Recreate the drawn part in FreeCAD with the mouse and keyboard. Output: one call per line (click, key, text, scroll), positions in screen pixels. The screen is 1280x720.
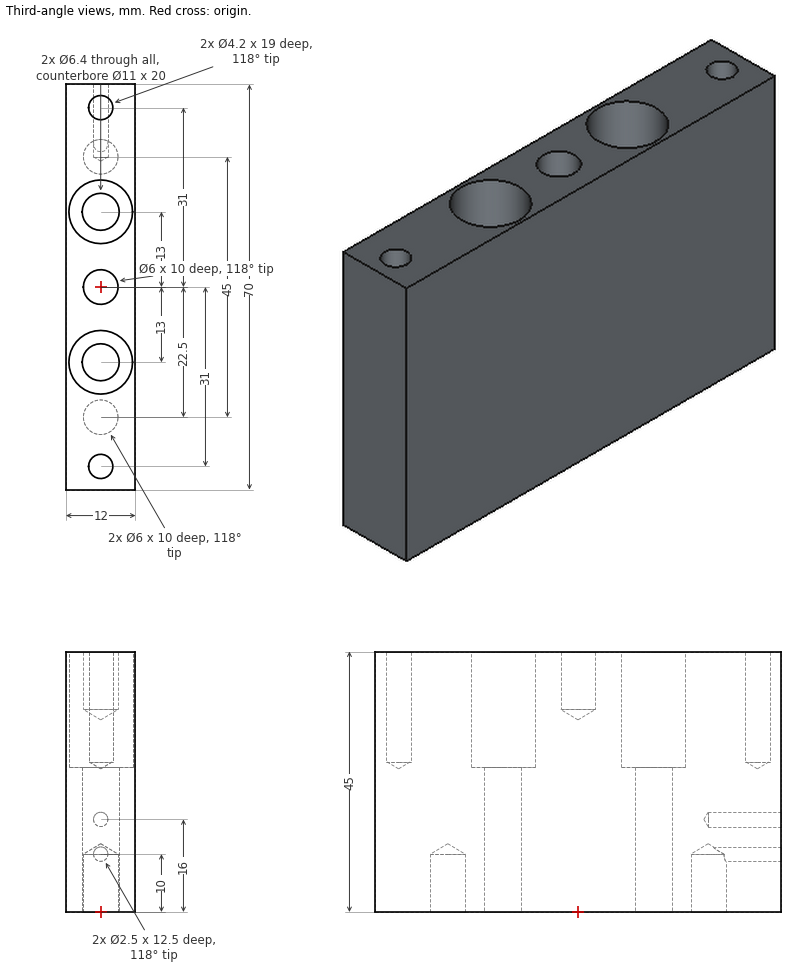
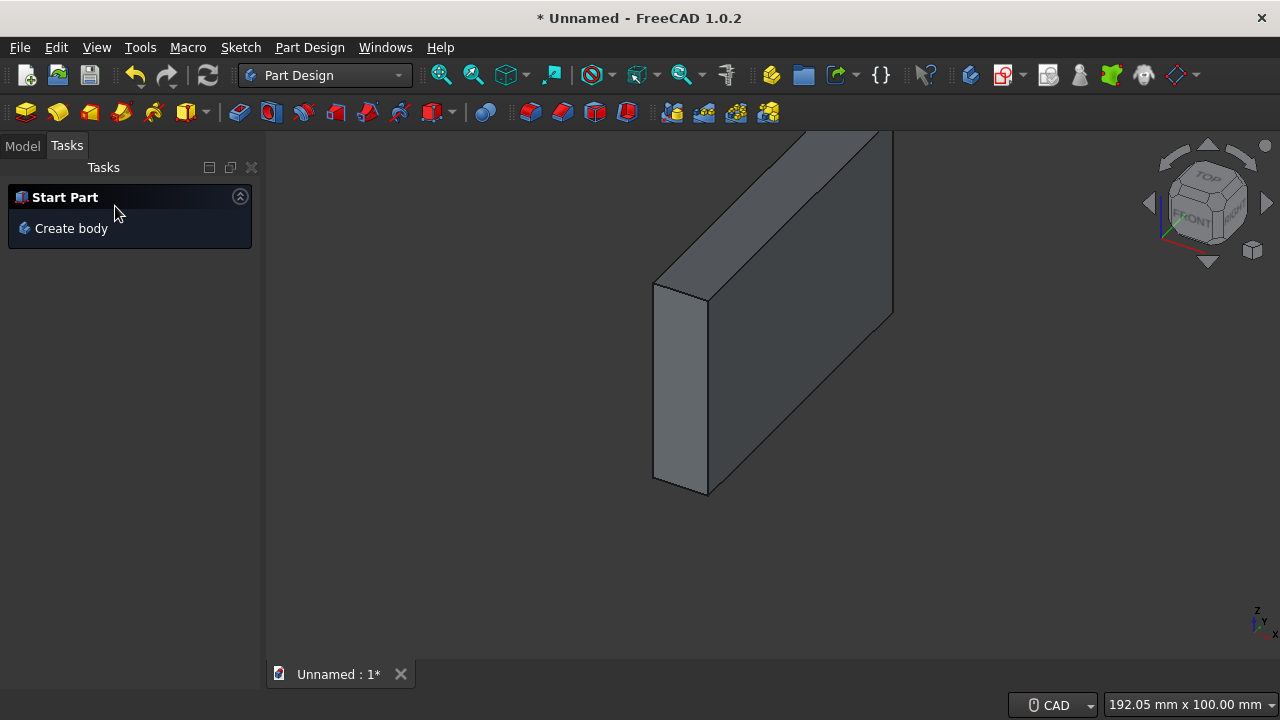
click(442, 76)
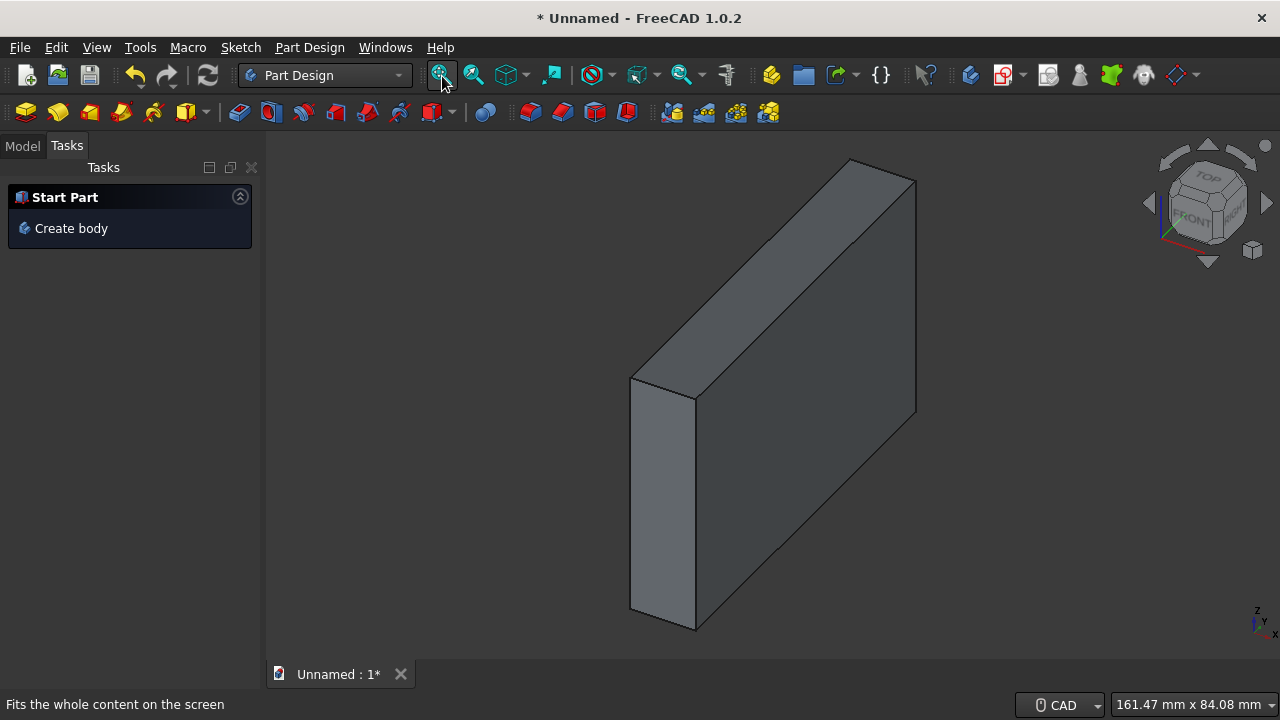
key(4)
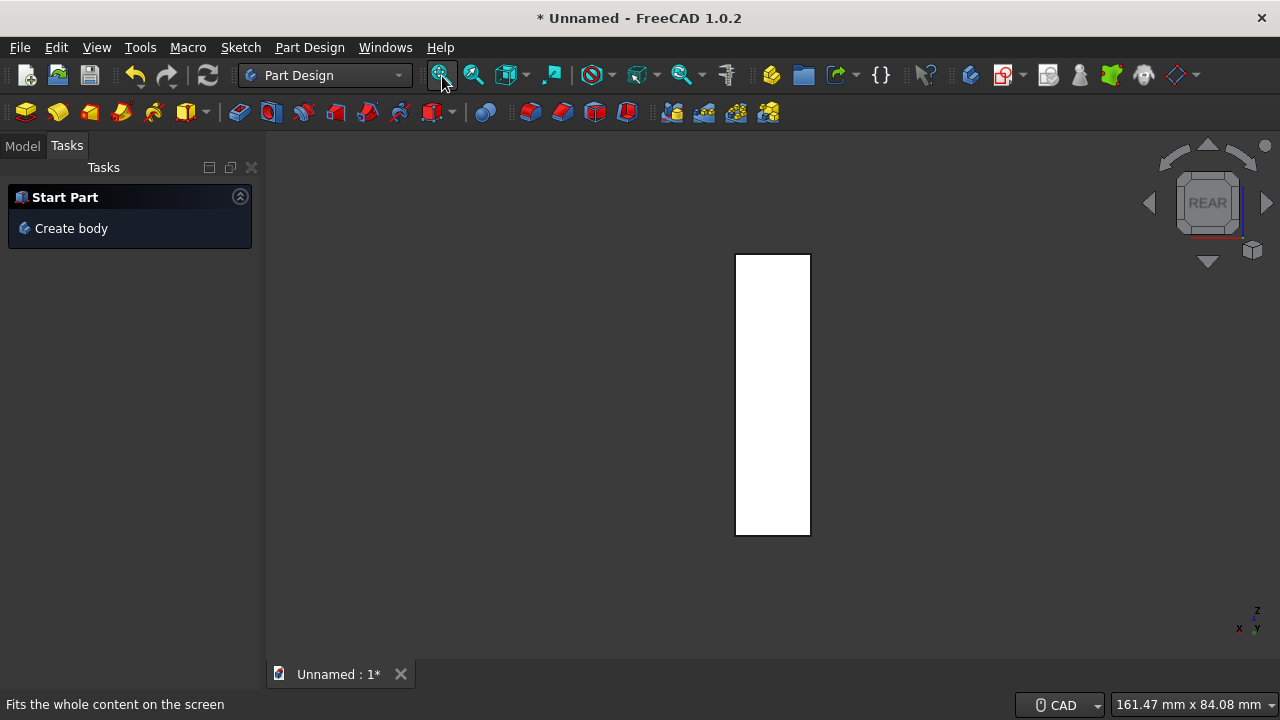
click(773, 313)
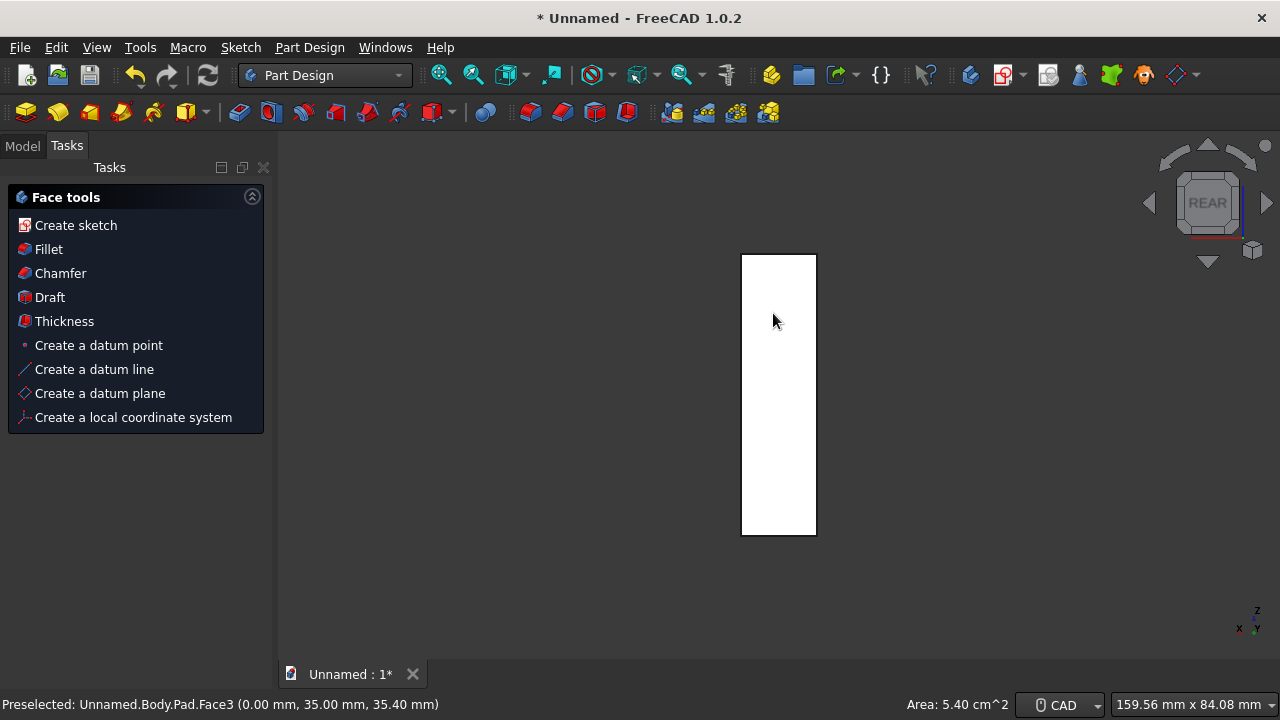
click(1004, 76)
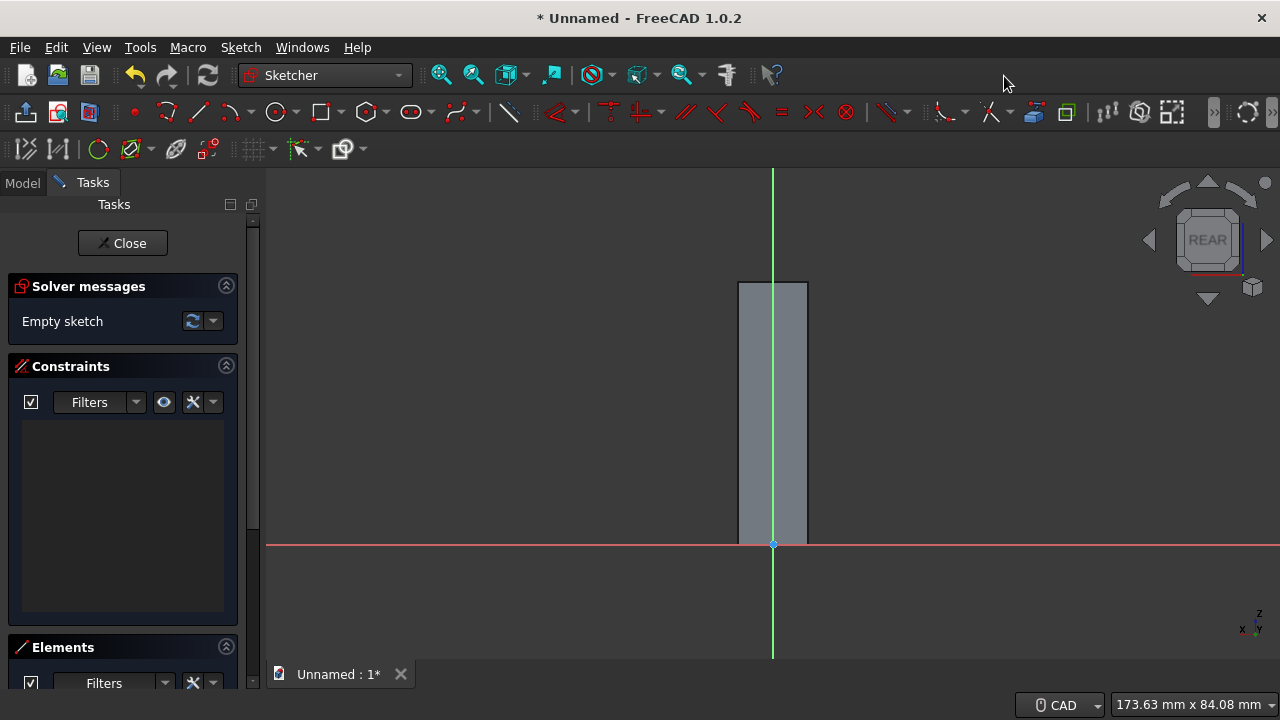
scroll(803, 529, up, 6)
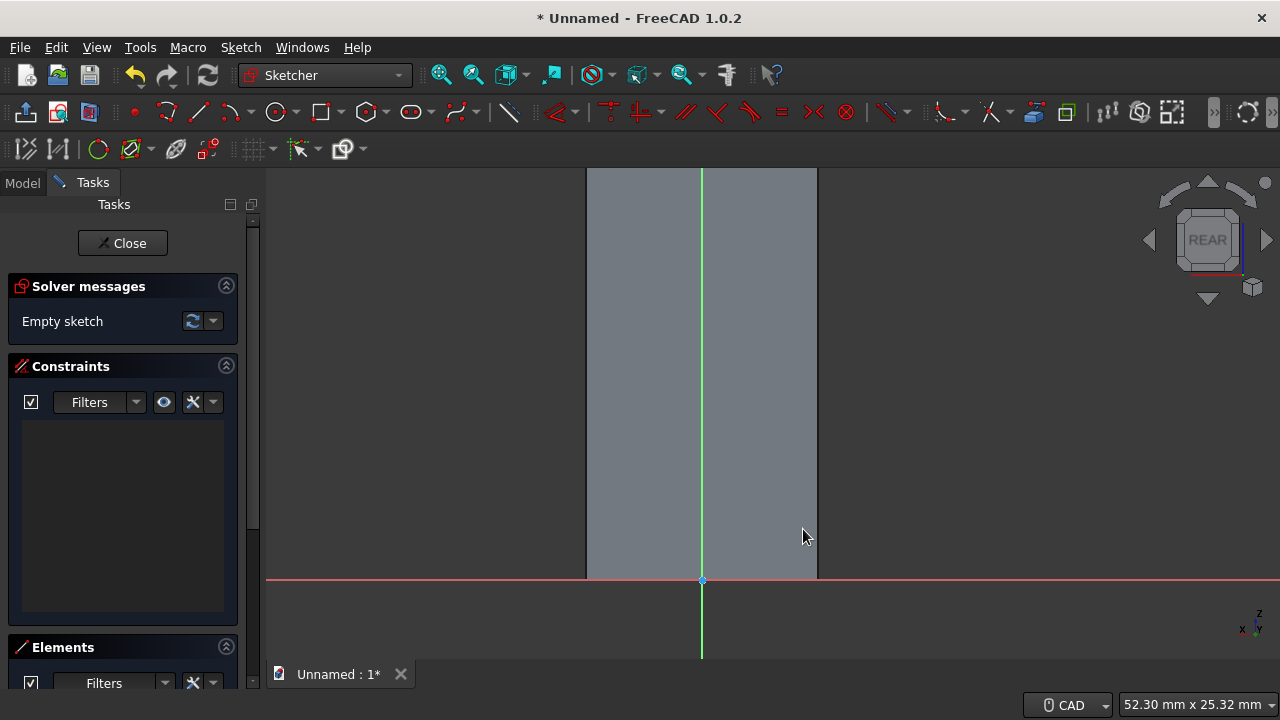
click(276, 112)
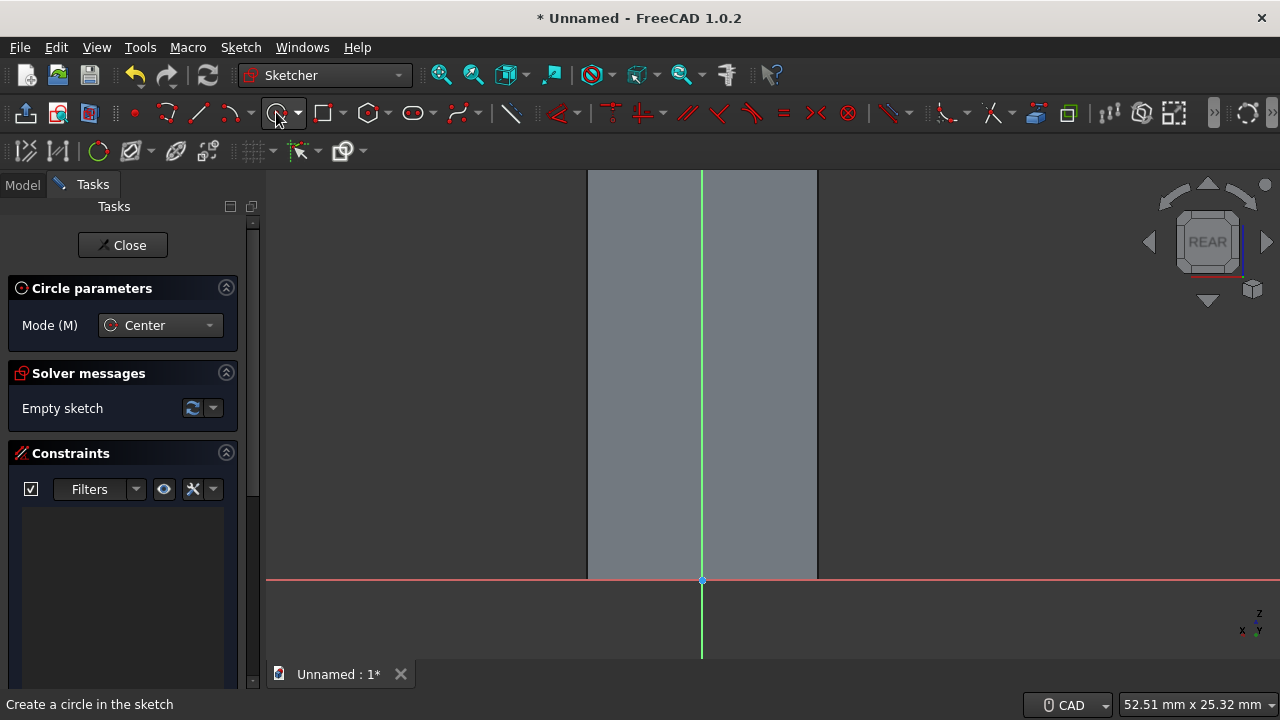
click(702, 387)
move(720, 370)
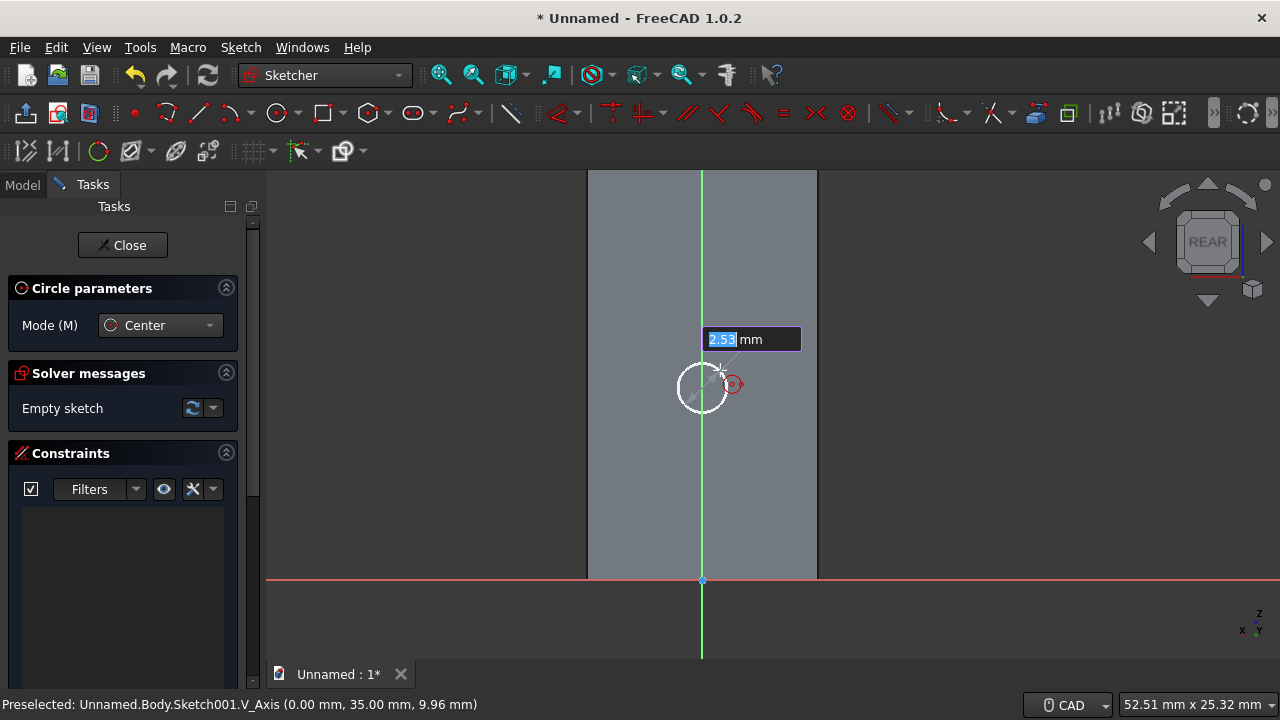
text(2.5)
key(Return)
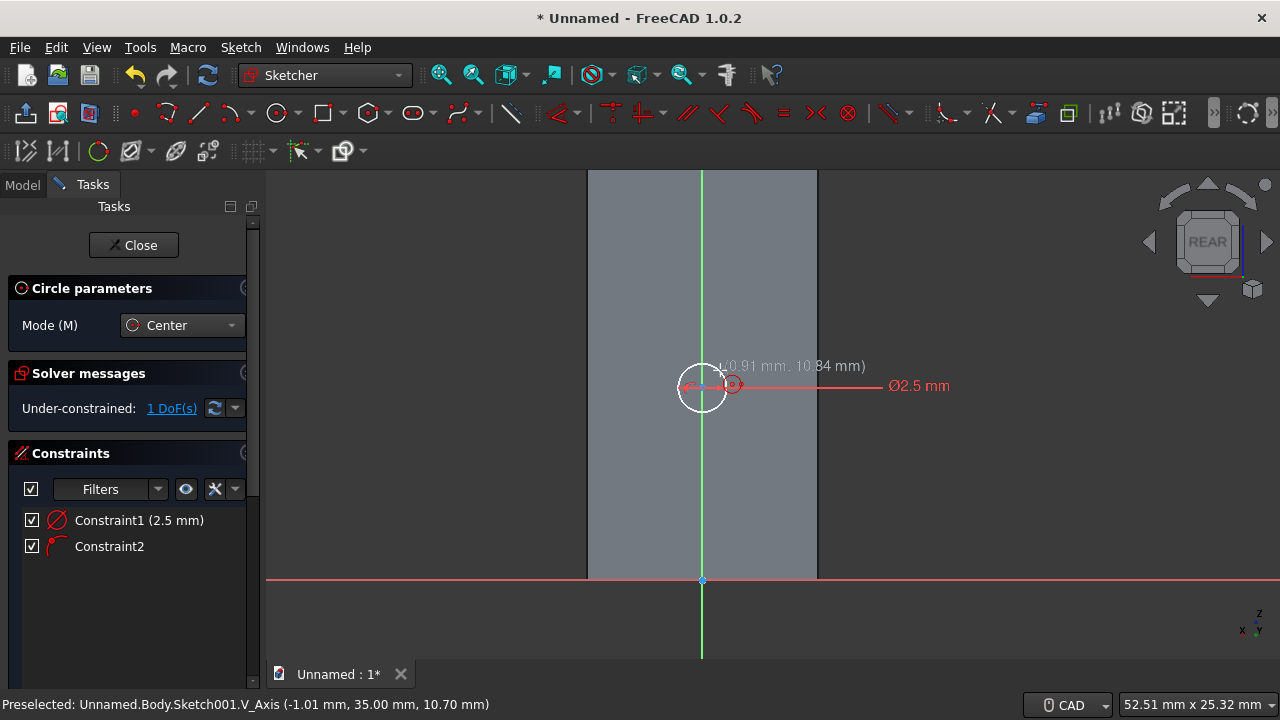
click(702, 271)
move(720, 254)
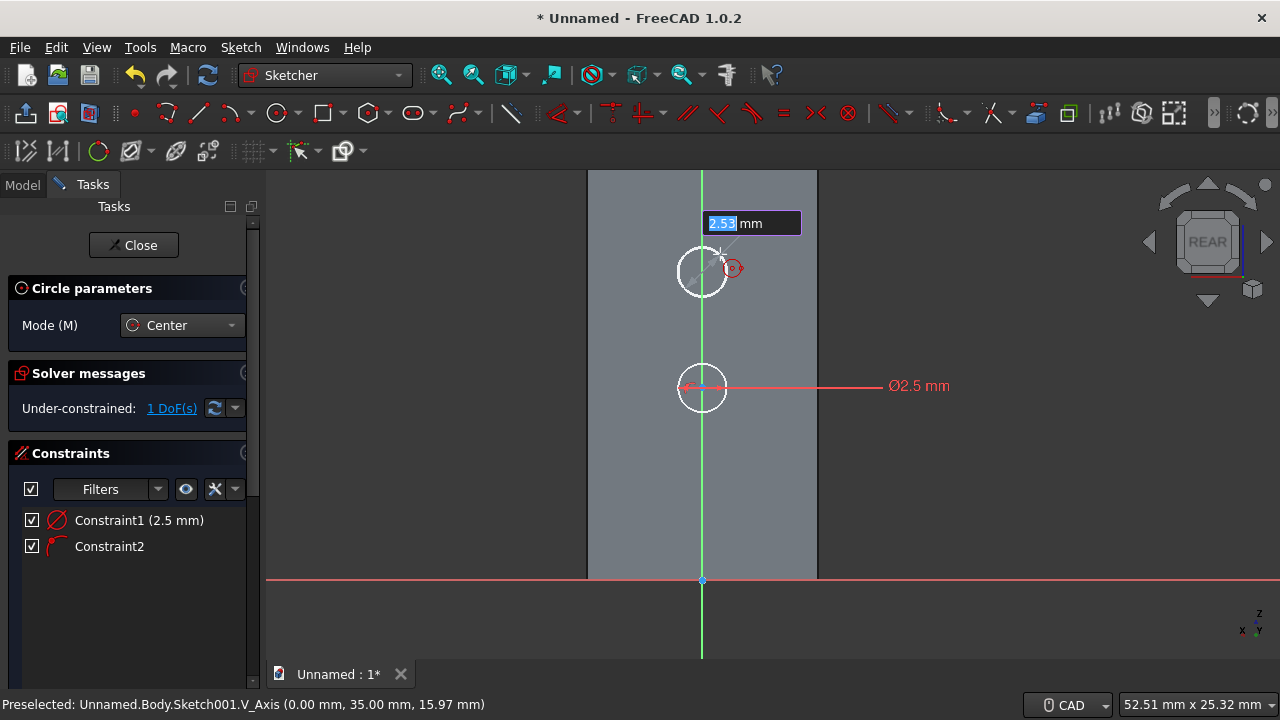
text(2.5)
key(Return)
key(Escape)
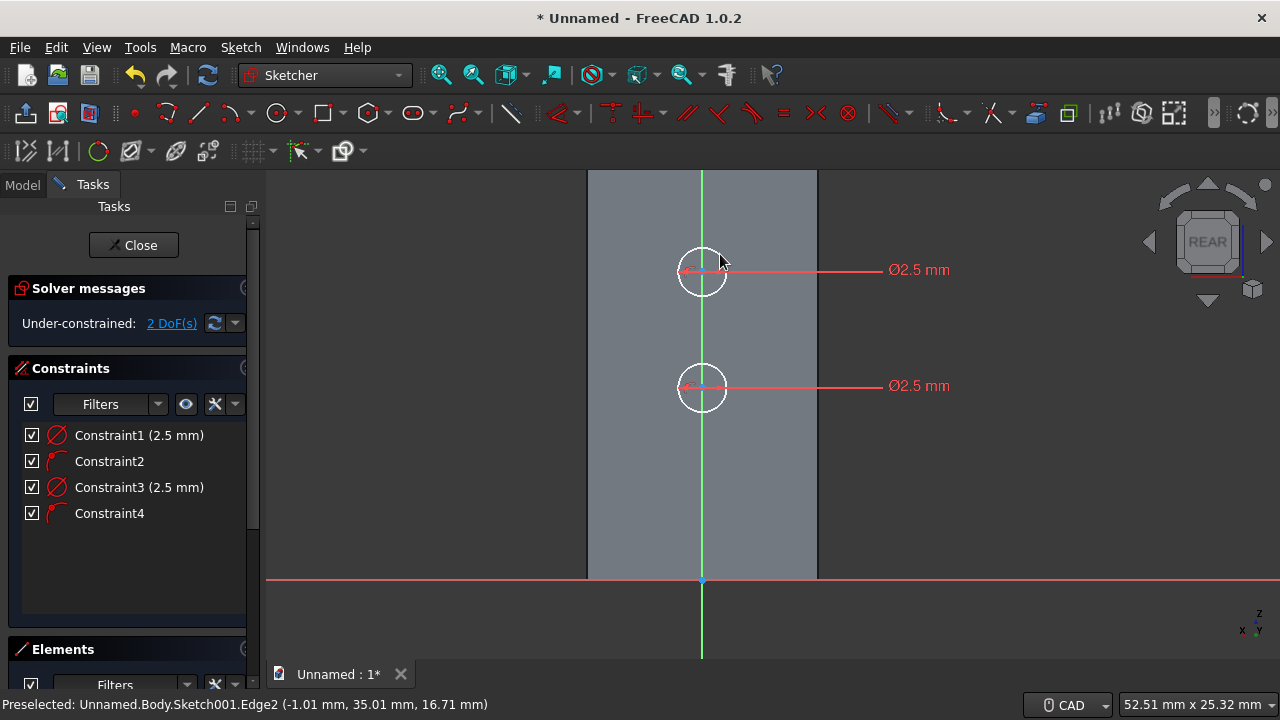
click(558, 114)